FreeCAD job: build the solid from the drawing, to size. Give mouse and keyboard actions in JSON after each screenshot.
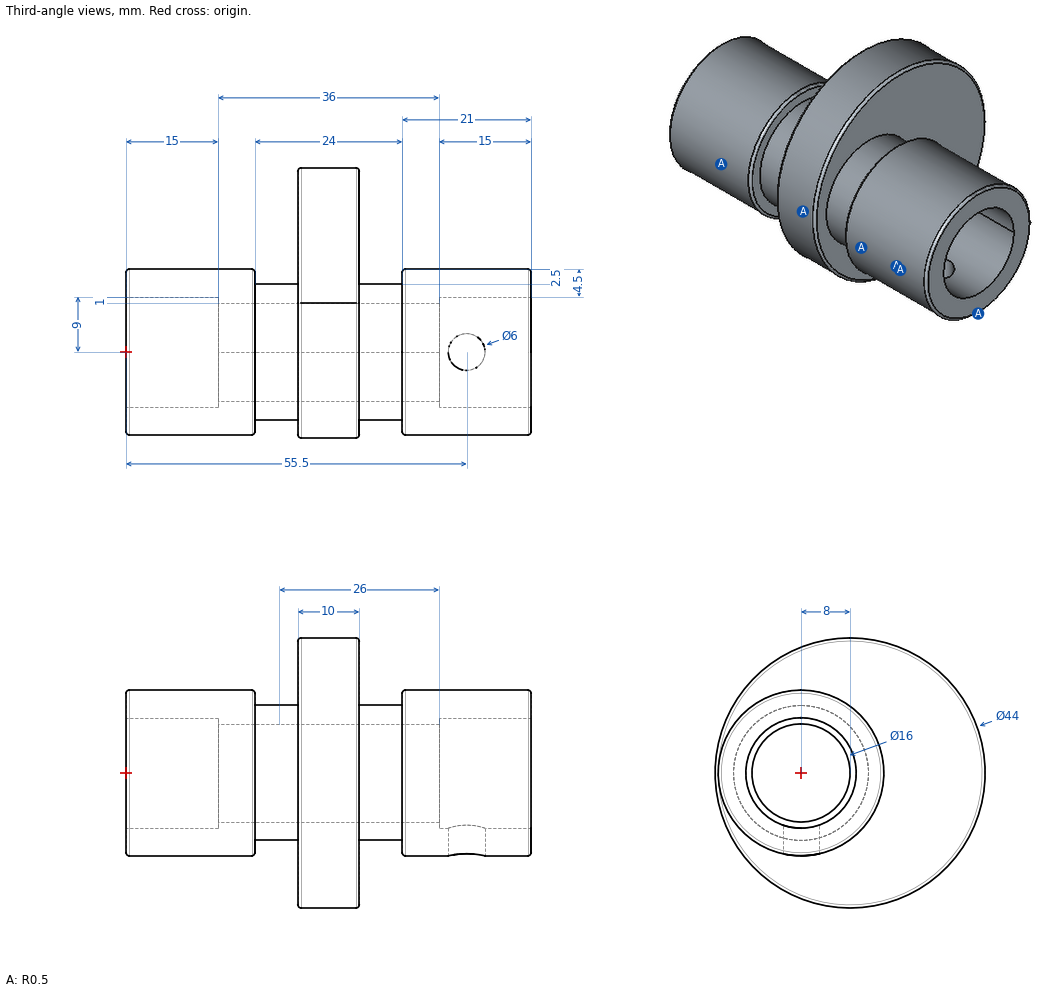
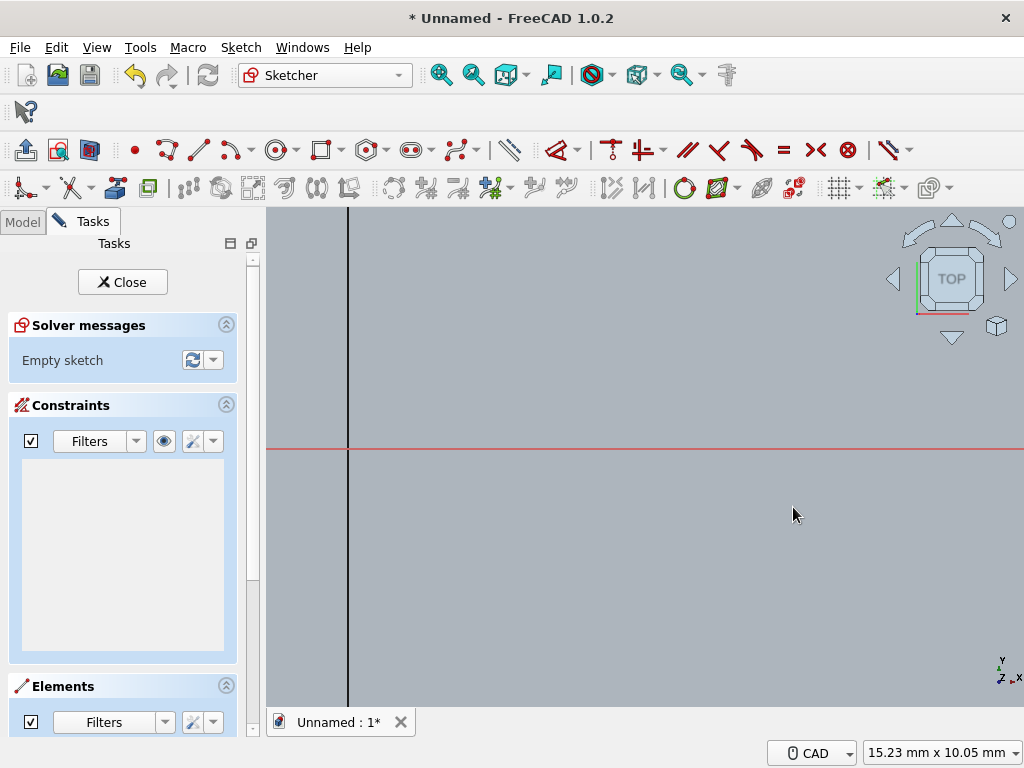
{"action": "left_click", "coordinate": [276, 150]}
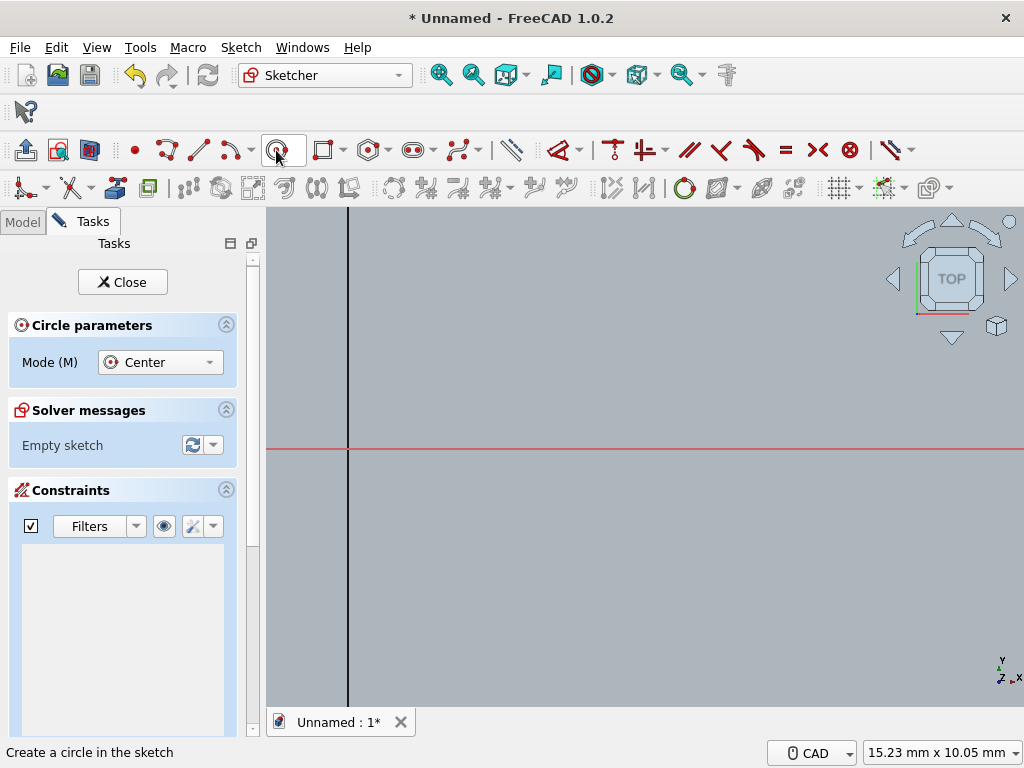
{"action": "left_click", "coordinate": [572, 449]}
{"action": "mouse_move", "coordinate": [677, 344]}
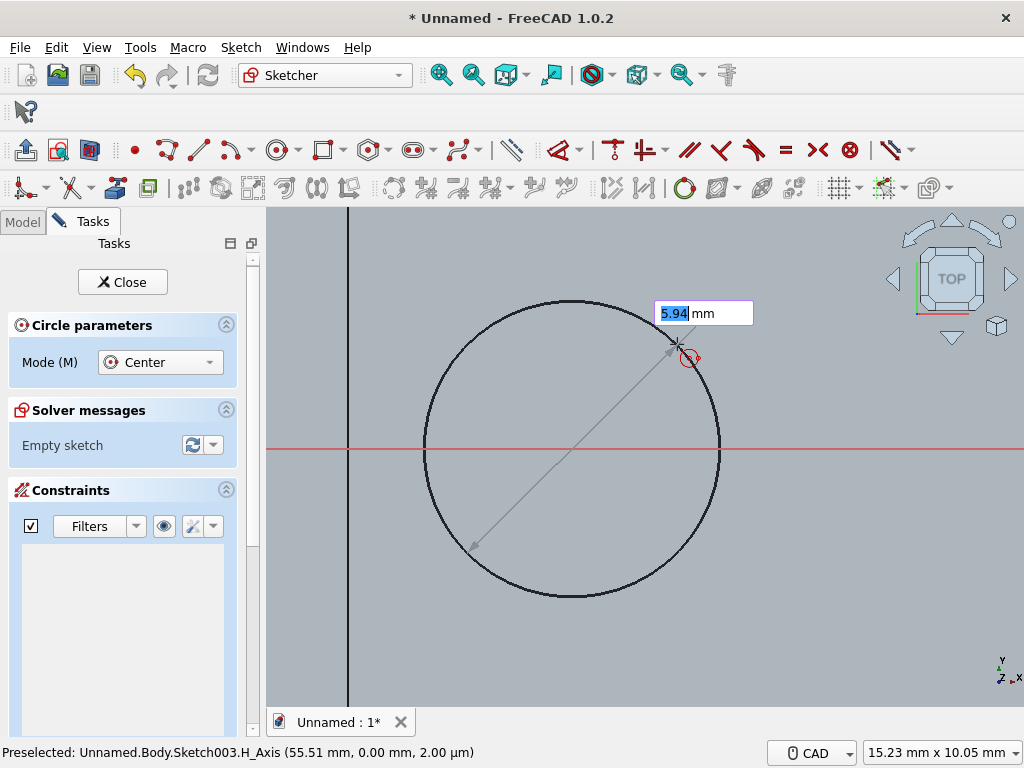
{"action": "type", "text": "6"}
{"action": "key", "text": "Return"}
{"action": "key", "text": "Escape"}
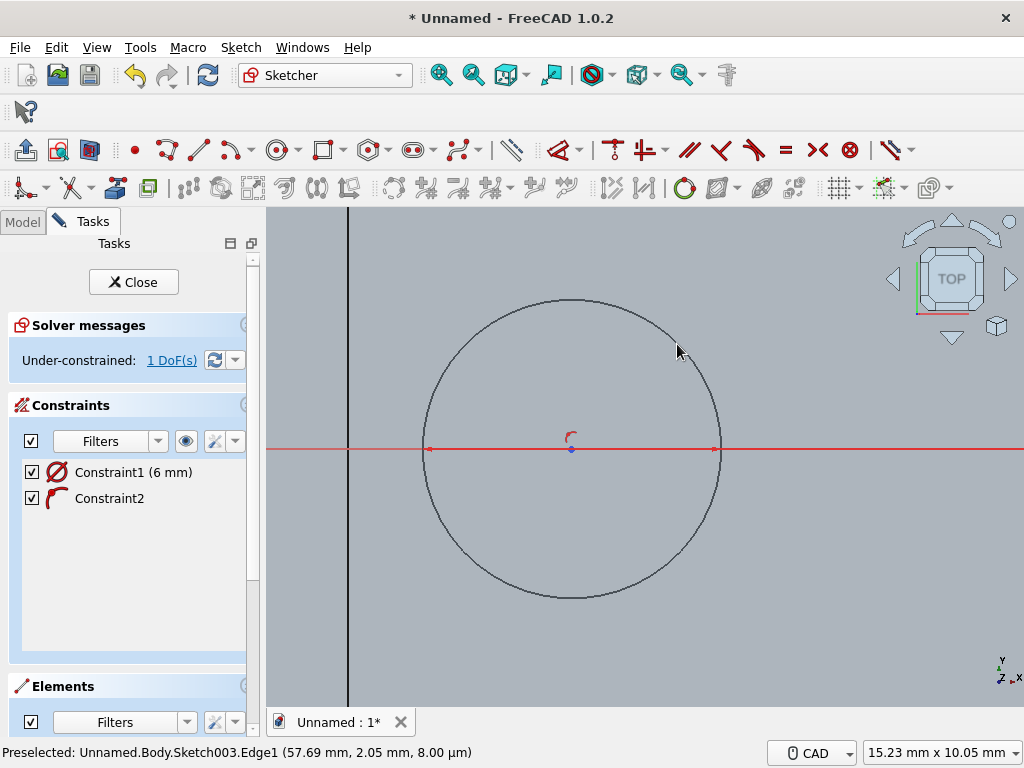
{"action": "left_click", "coordinate": [558, 150]}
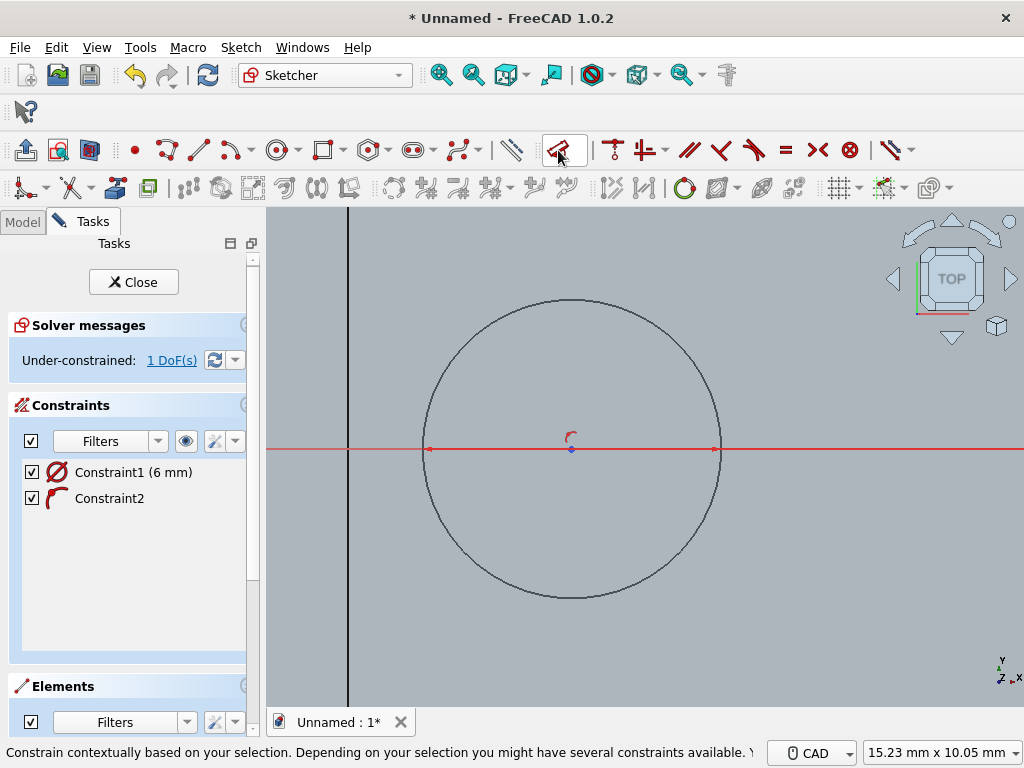
{"action": "left_click", "coordinate": [572, 449]}
{"action": "left_click", "coordinate": [369, 483]}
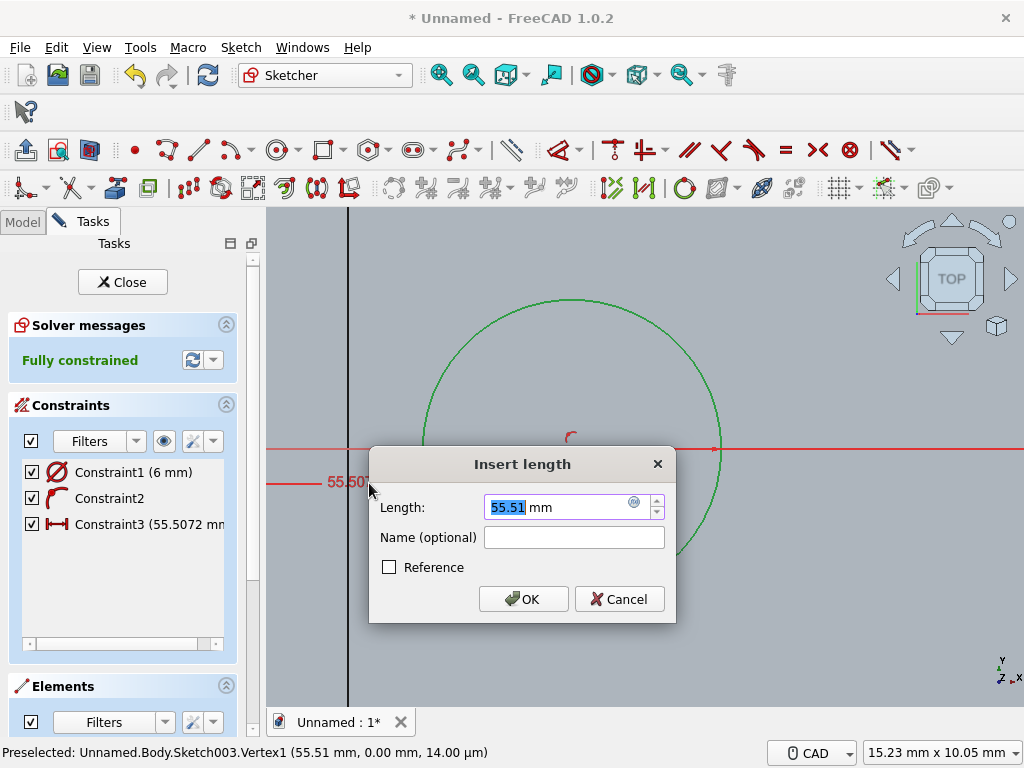
{"action": "type", "text": "55.5"}
{"action": "key", "text": "Return"}
{"action": "key", "text": "Escape"}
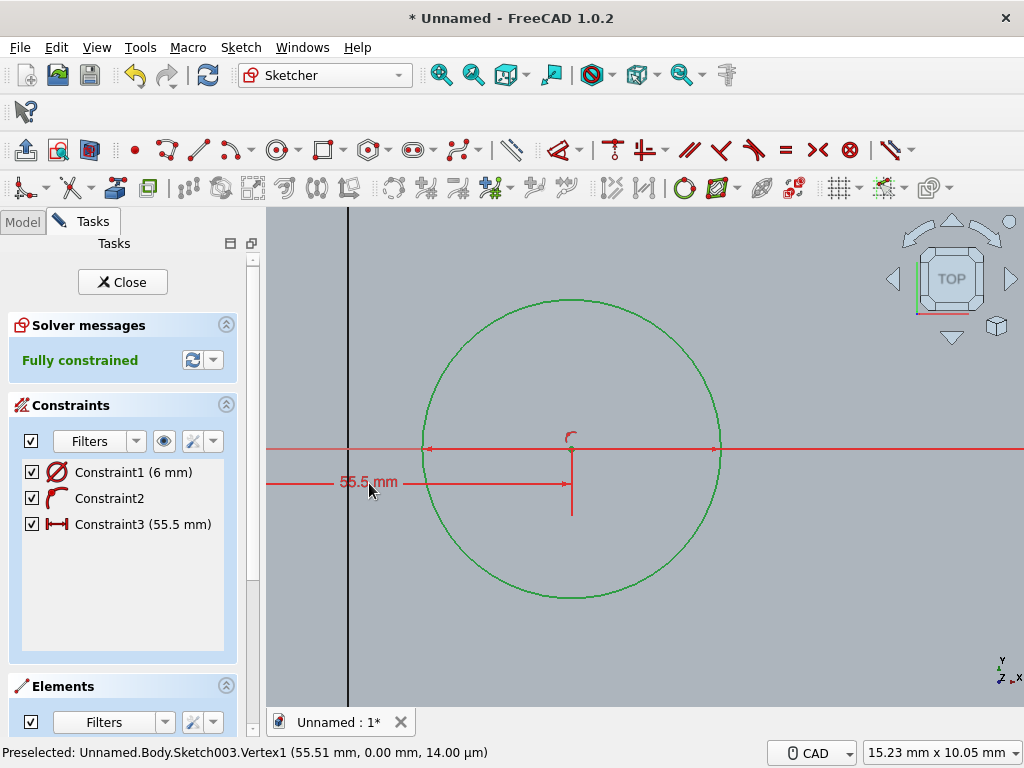
{"action": "left_click", "coordinate": [123, 282]}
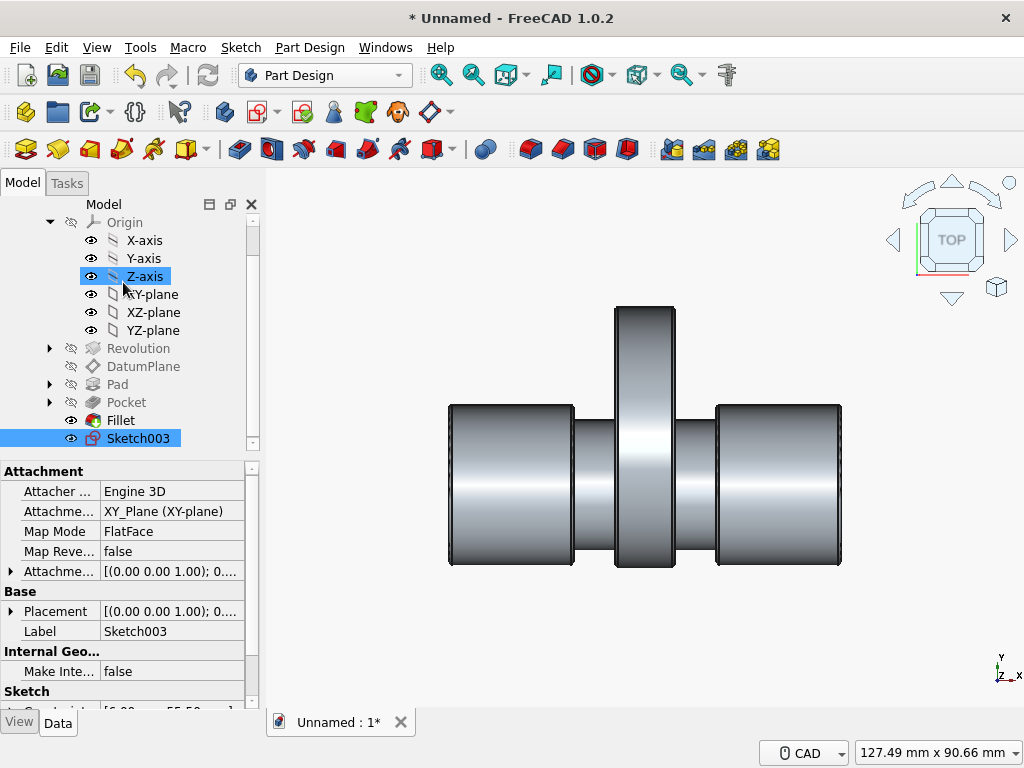
{"action": "left_click", "coordinate": [240, 150]}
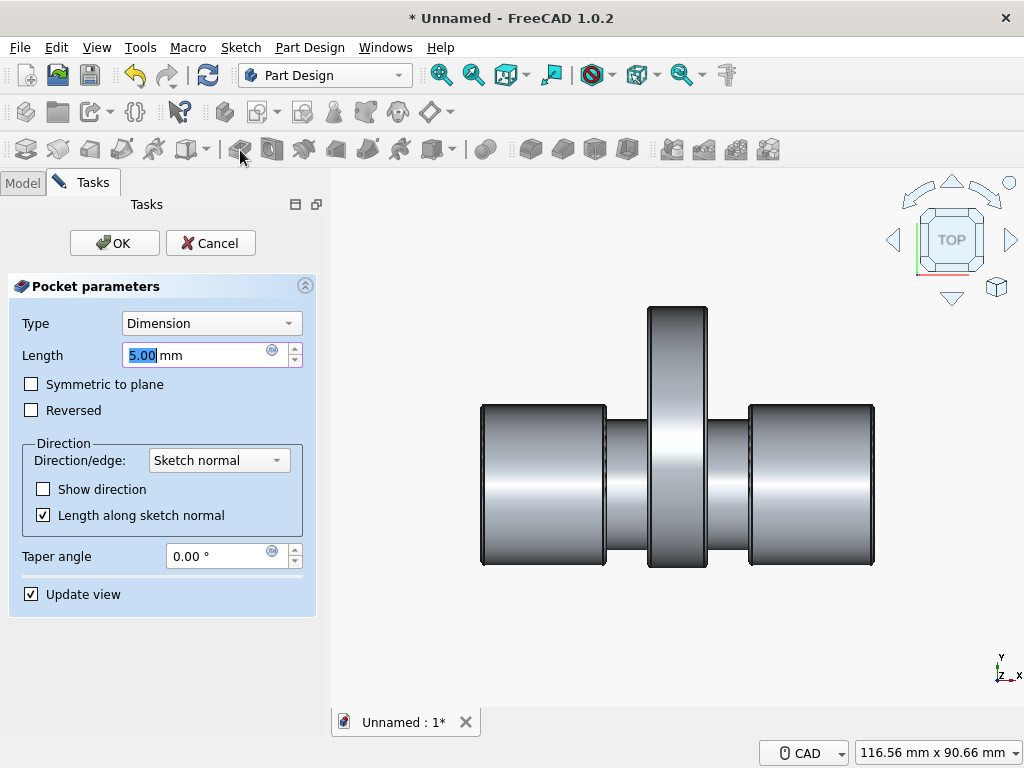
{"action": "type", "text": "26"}
{"action": "key", "text": "Tab"}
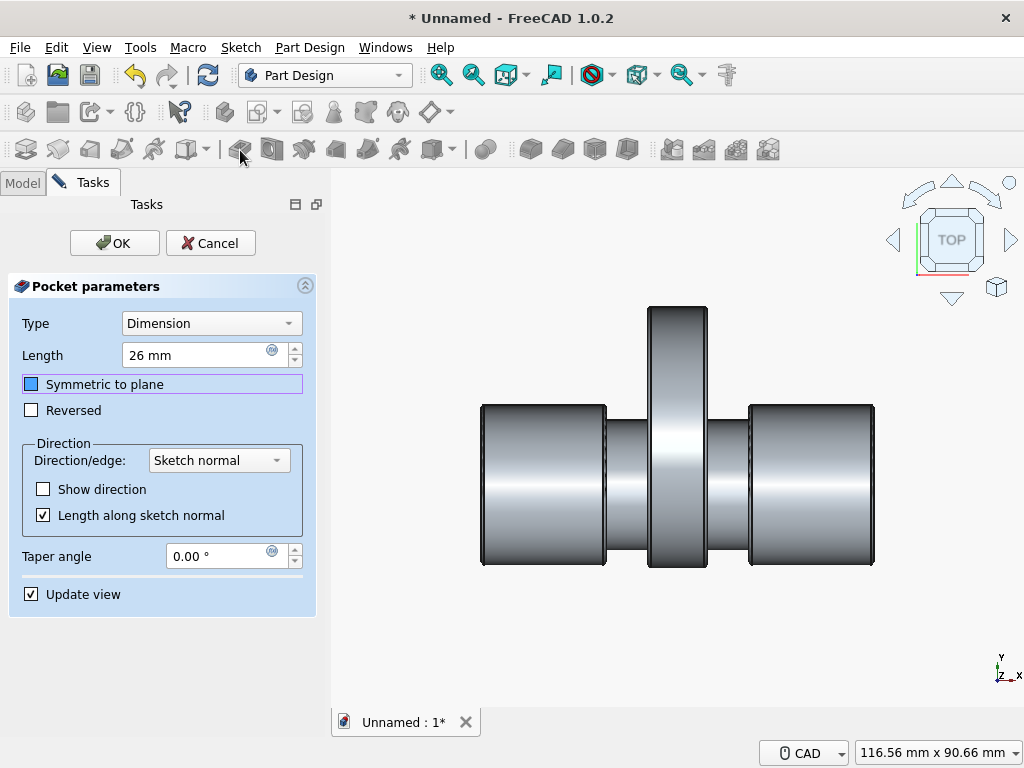
{"action": "left_click", "coordinate": [115, 243]}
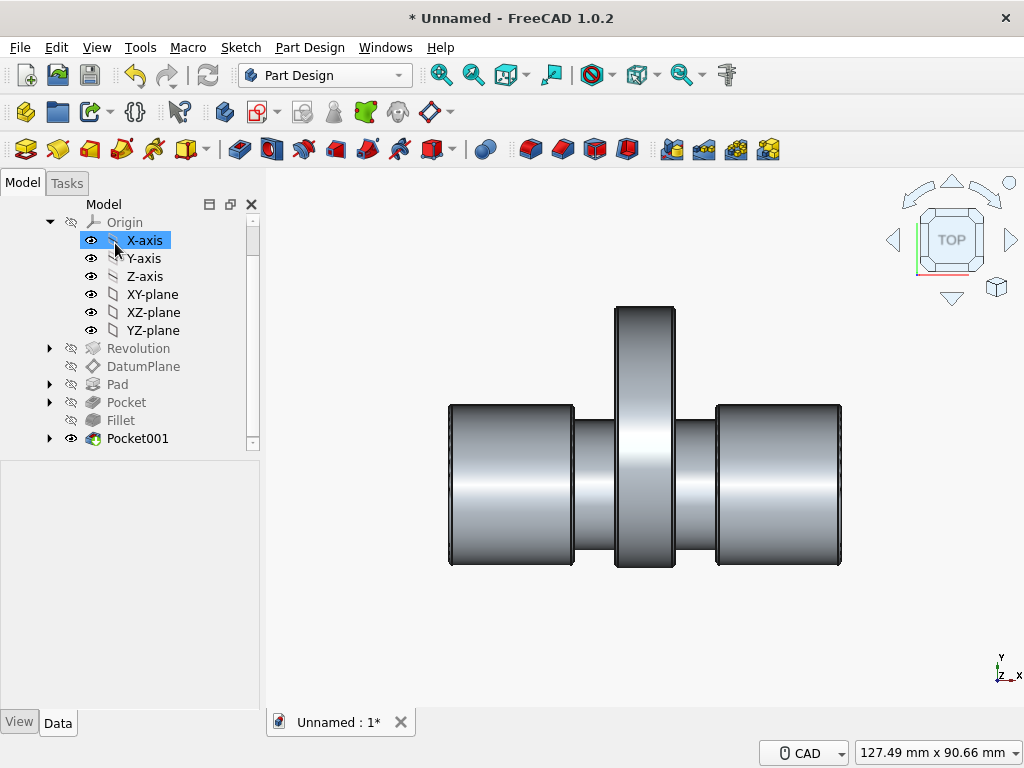
{"action": "key", "text": "0"}